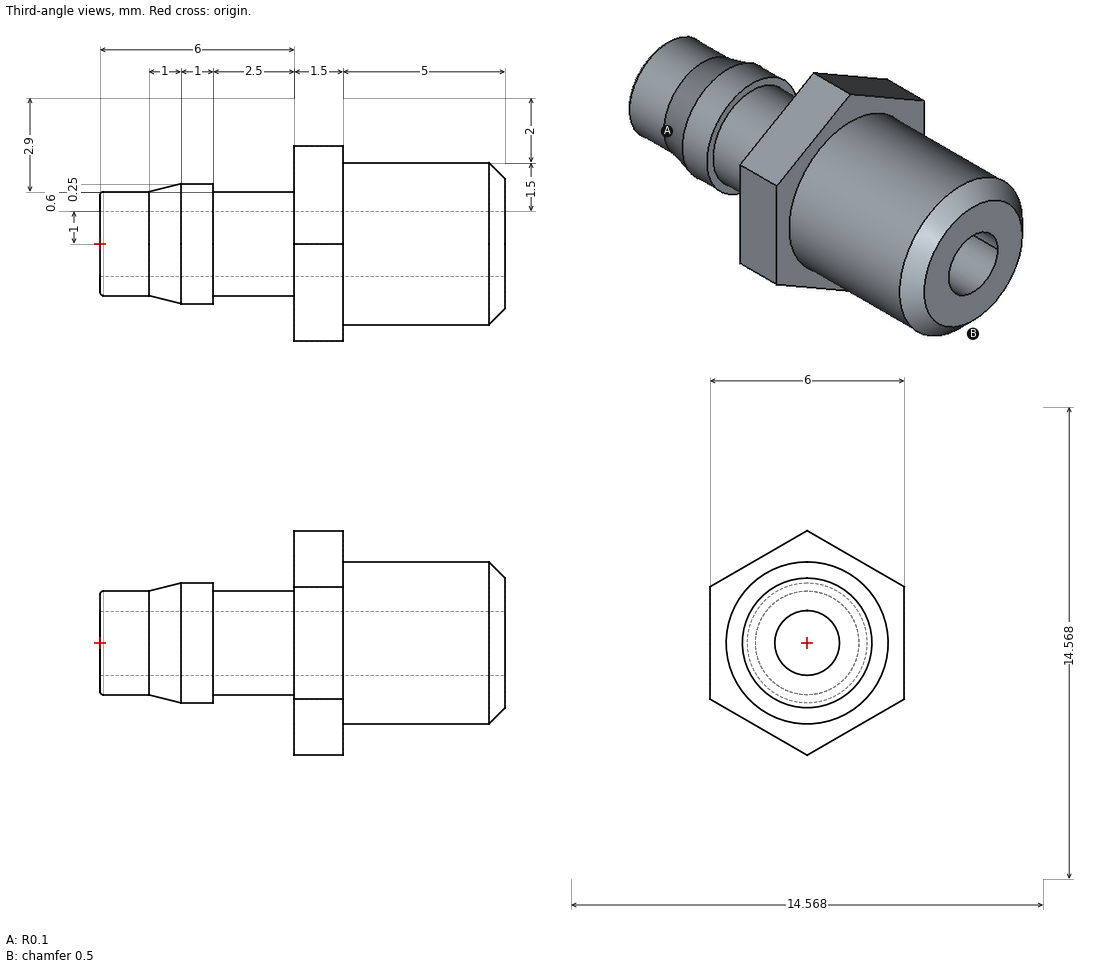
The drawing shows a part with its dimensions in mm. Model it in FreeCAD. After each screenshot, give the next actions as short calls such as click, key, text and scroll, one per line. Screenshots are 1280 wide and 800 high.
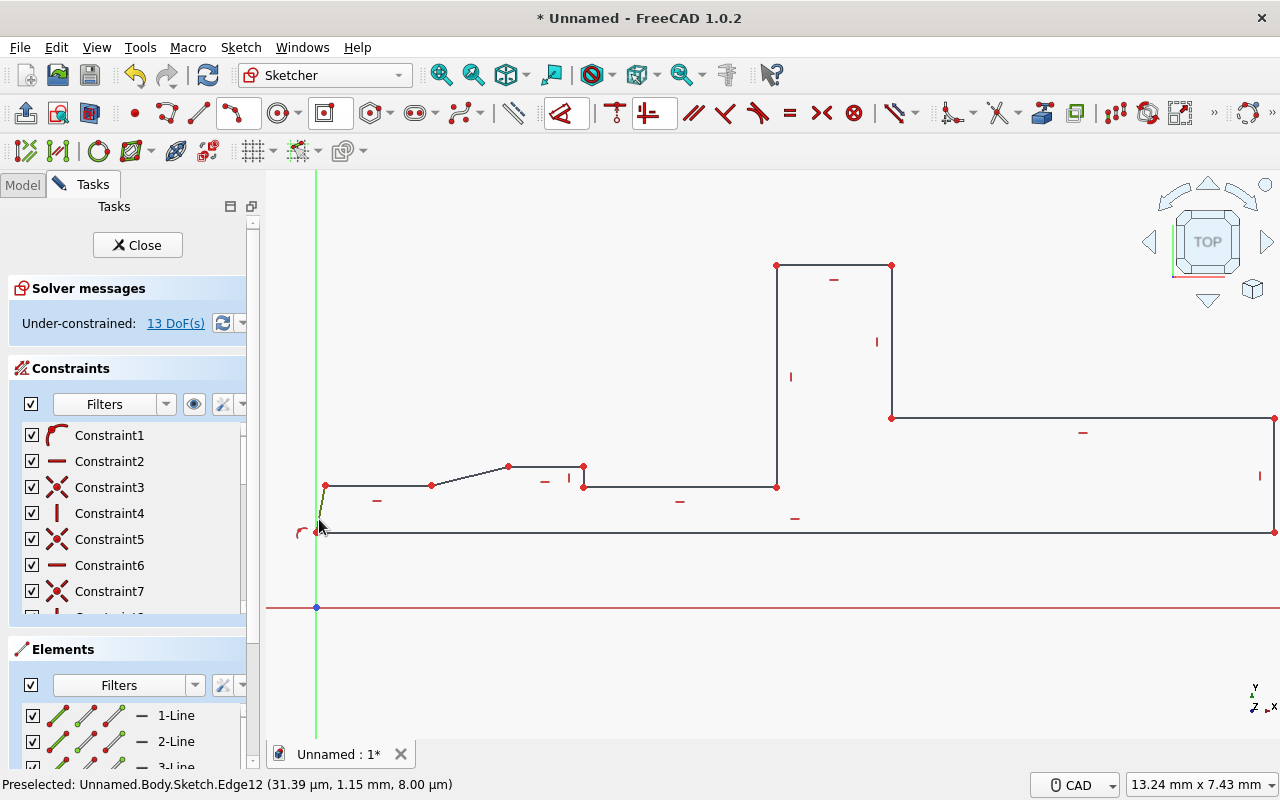
key(v)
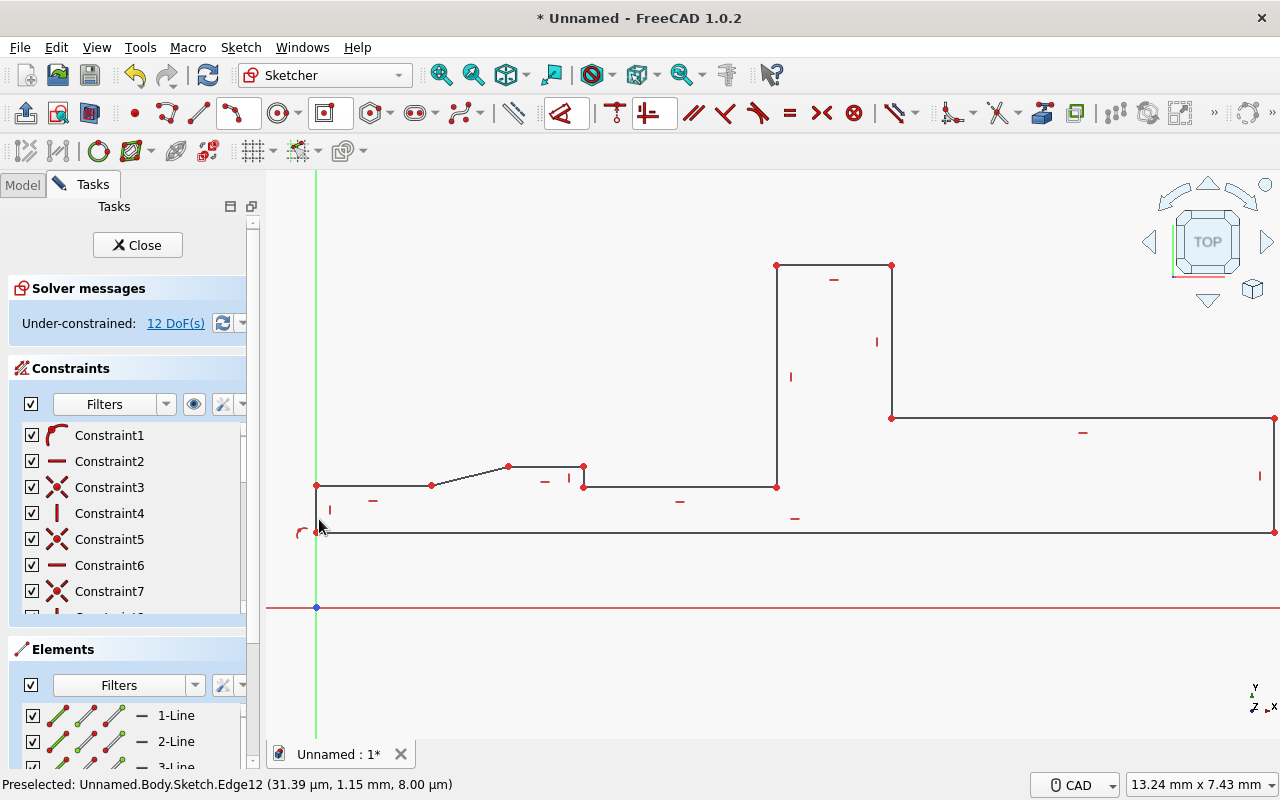
click(560, 114)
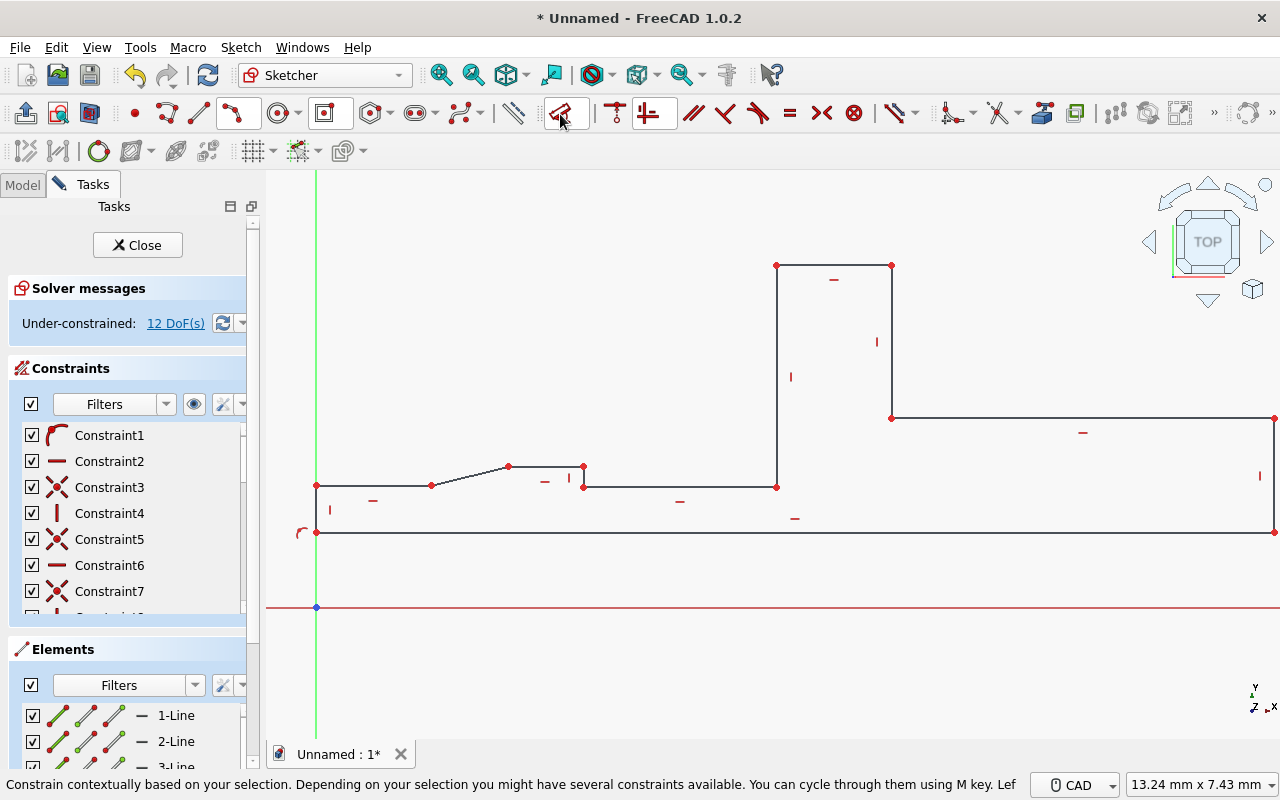
click(1006, 418)
click(1003, 384)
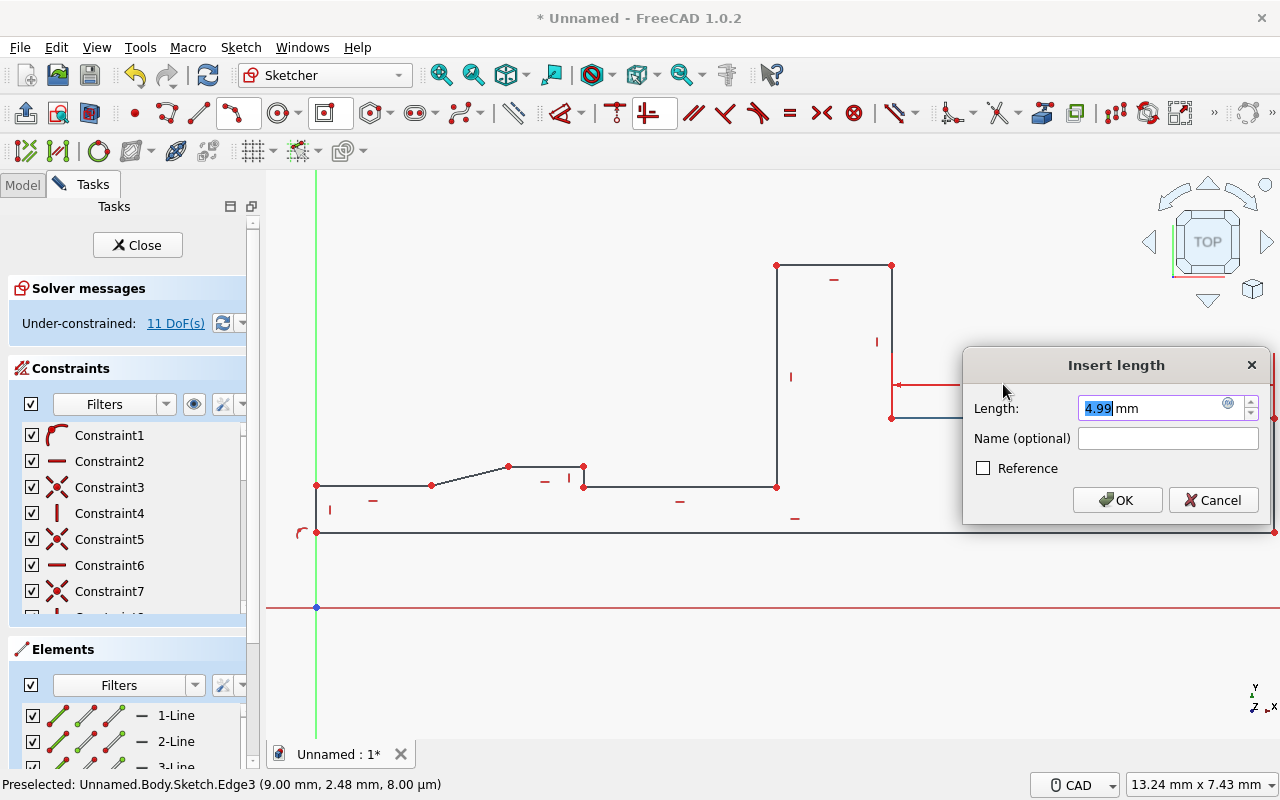
text(5)
key(Return)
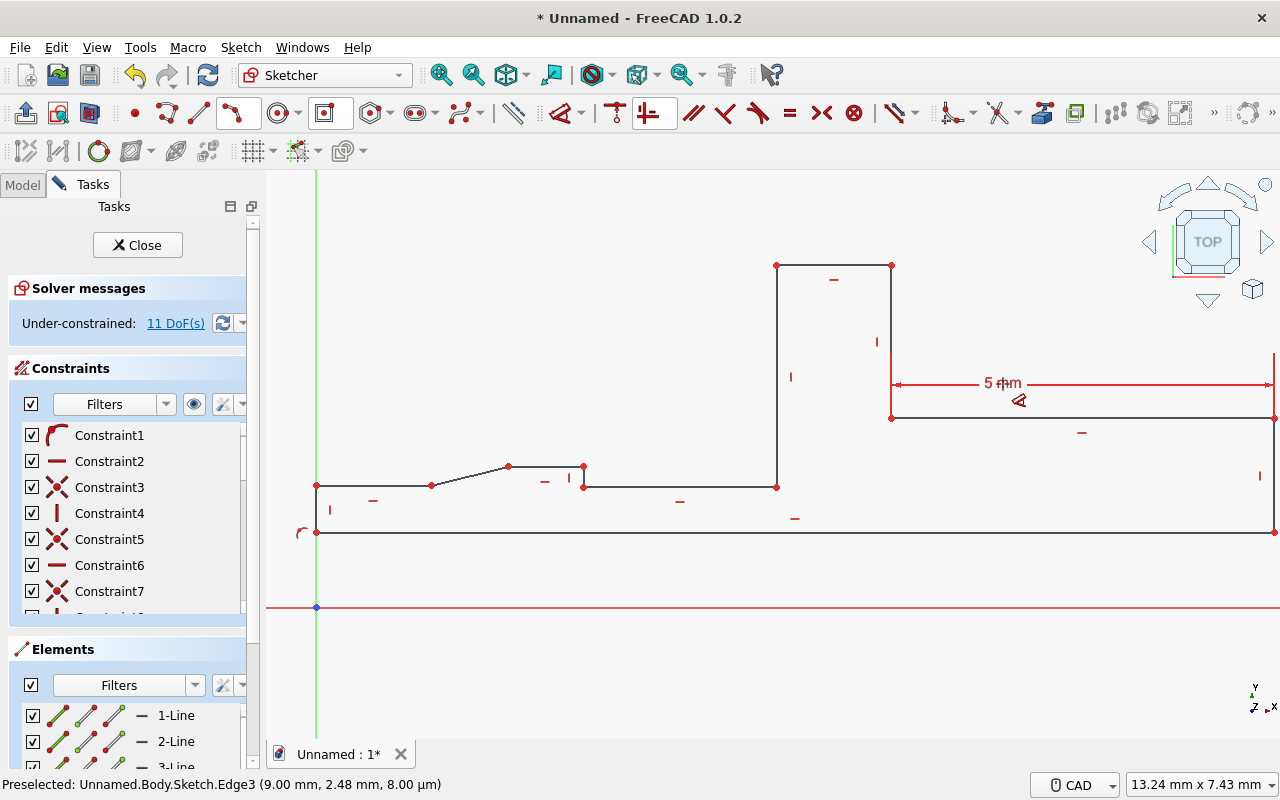
click(891, 372)
click(925, 342)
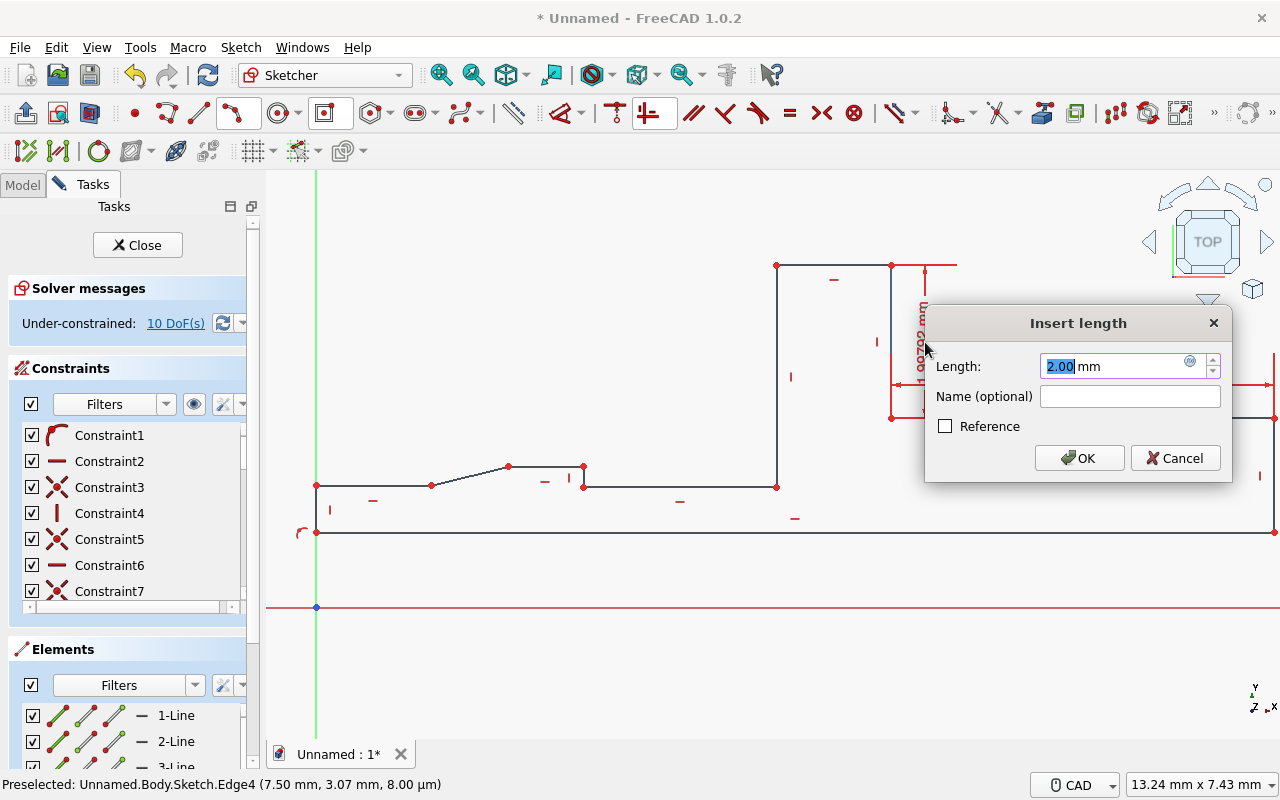
text(2)
key(Return)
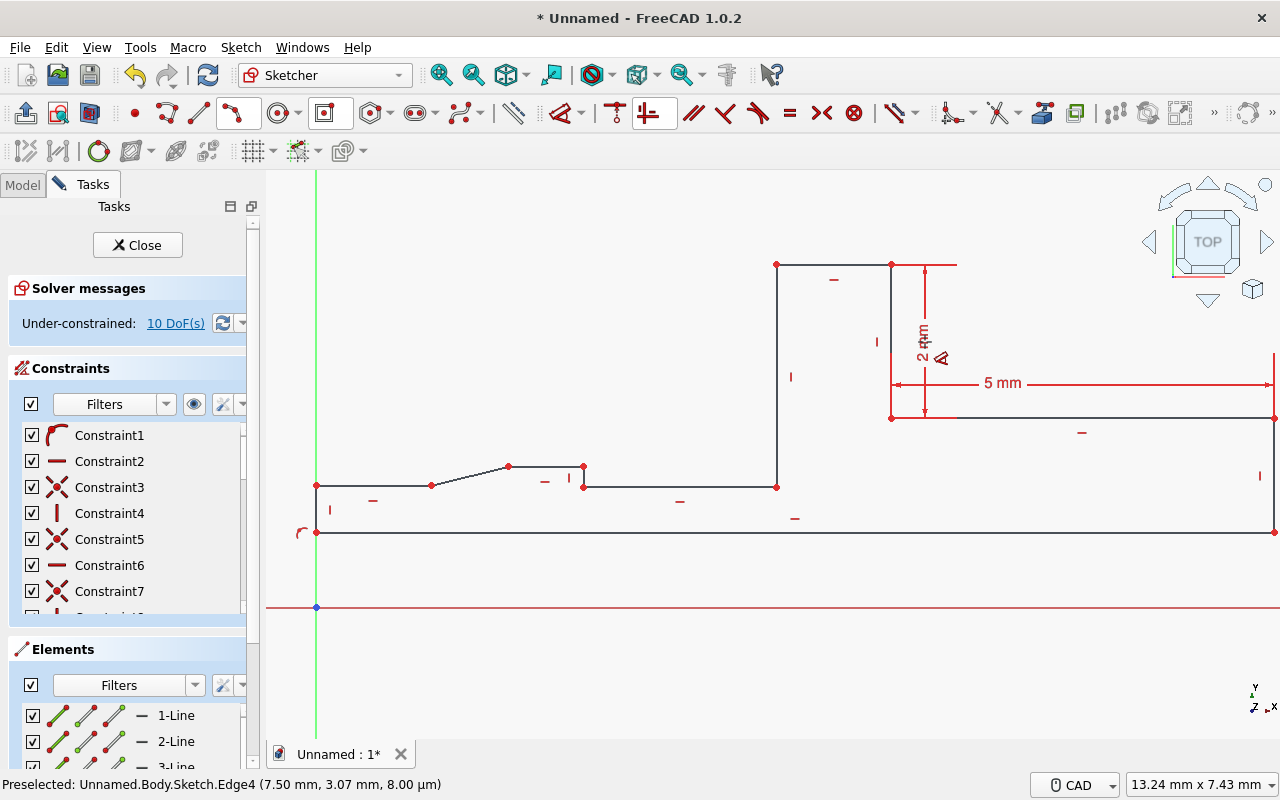
click(561, 467)
click(546, 501)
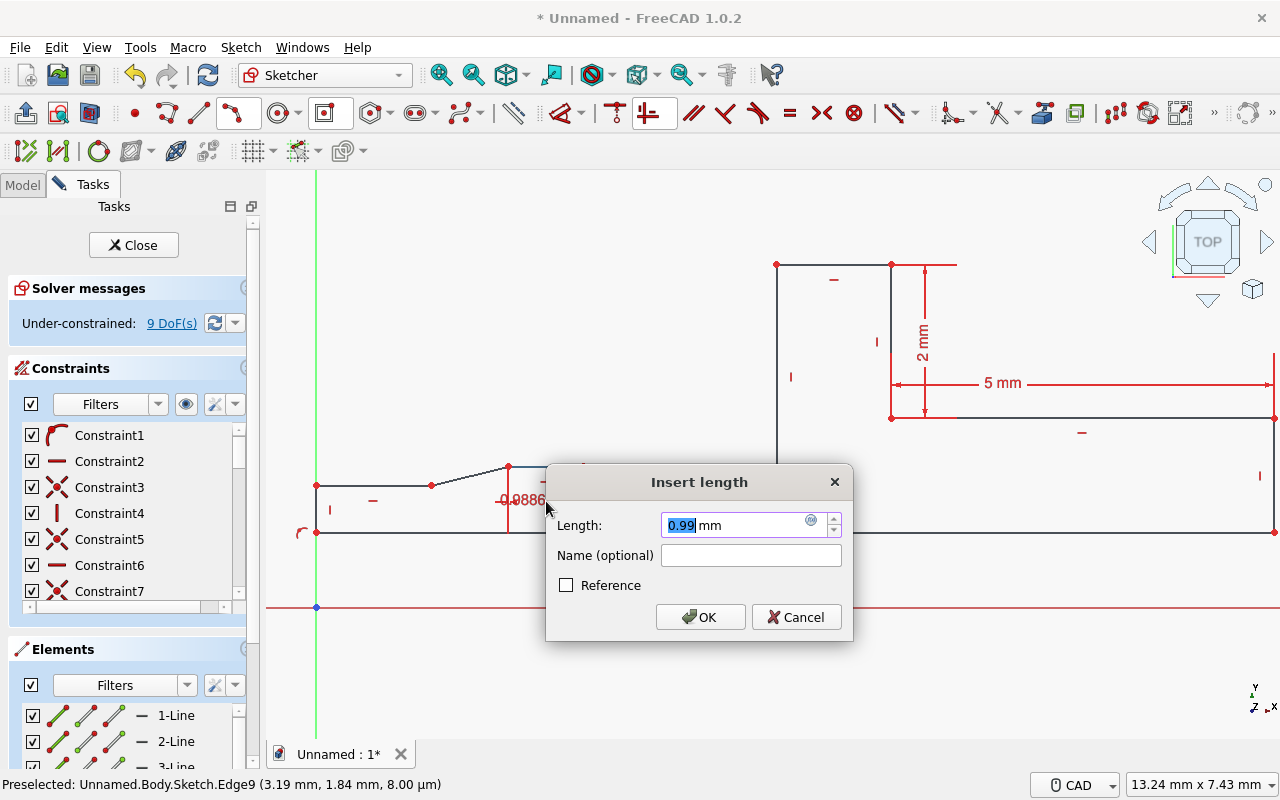
text(1)
key(Return)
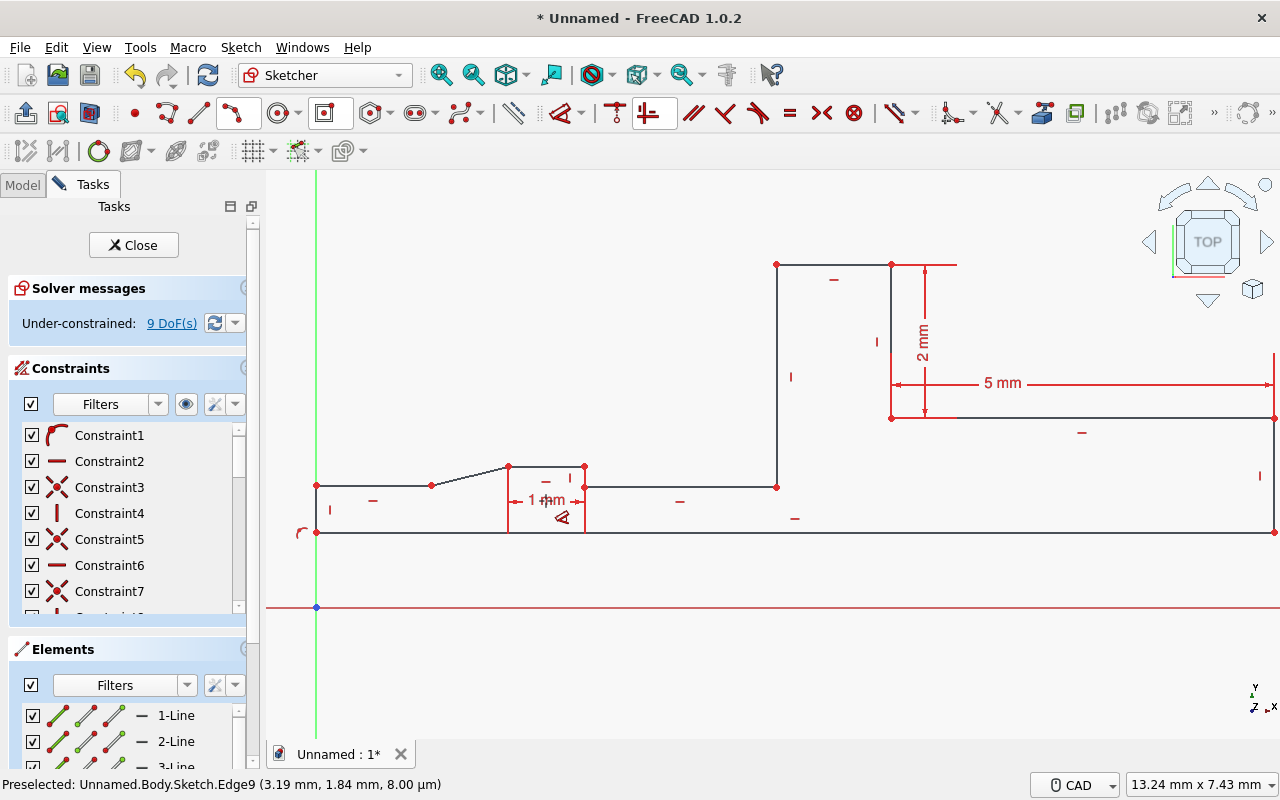
click(316, 533)
click(350, 570)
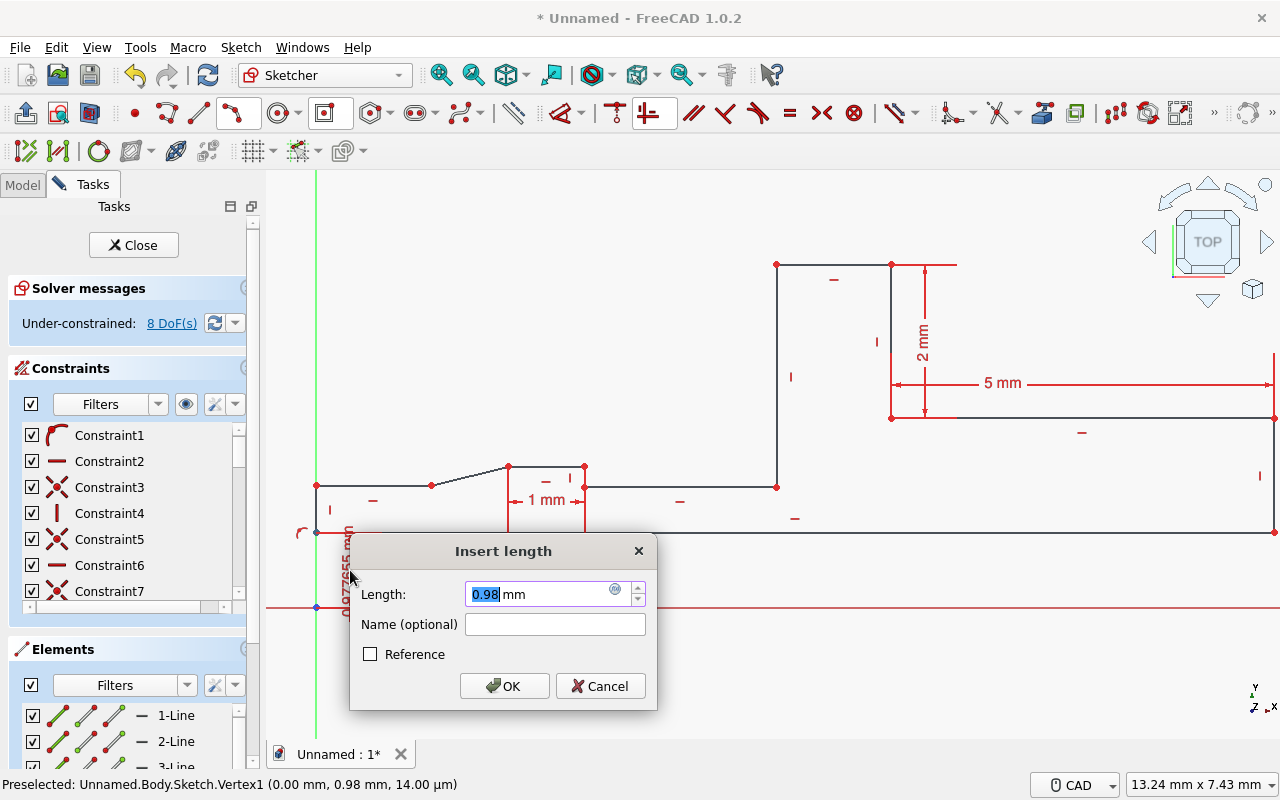
text(1)
key(Return)